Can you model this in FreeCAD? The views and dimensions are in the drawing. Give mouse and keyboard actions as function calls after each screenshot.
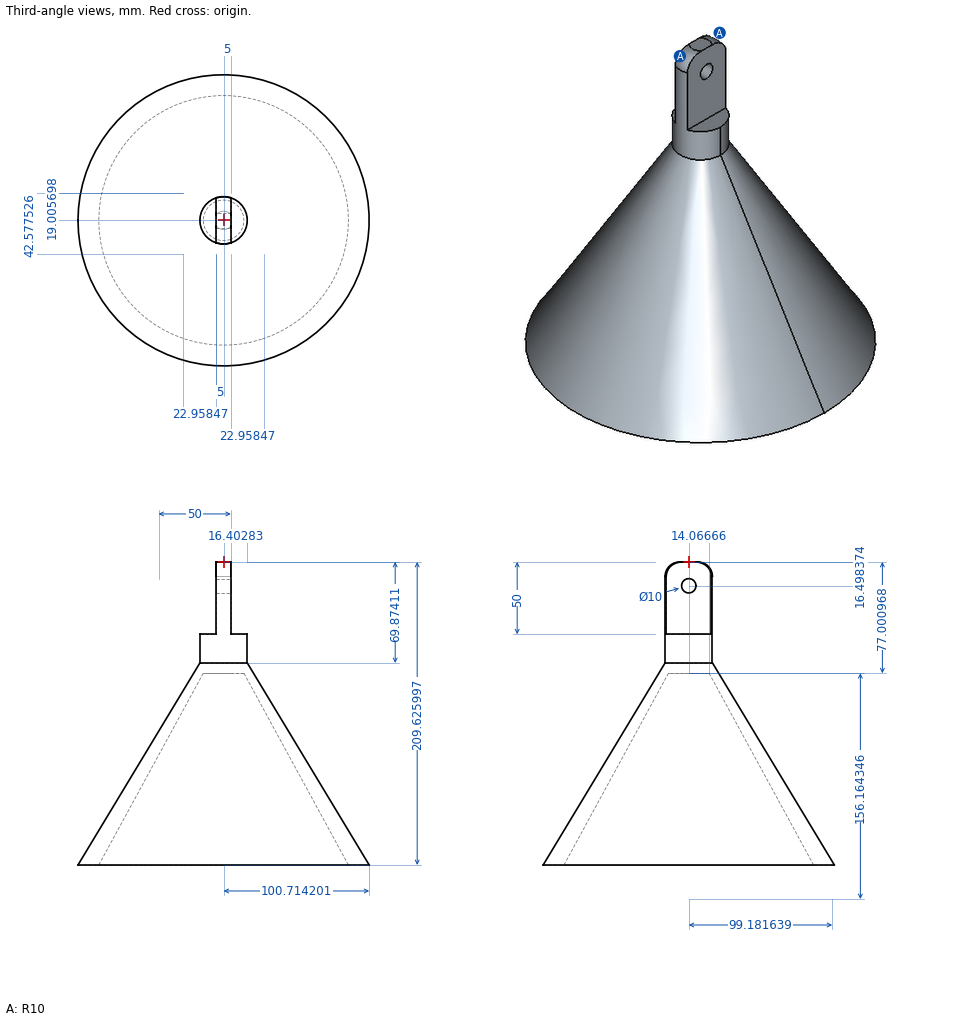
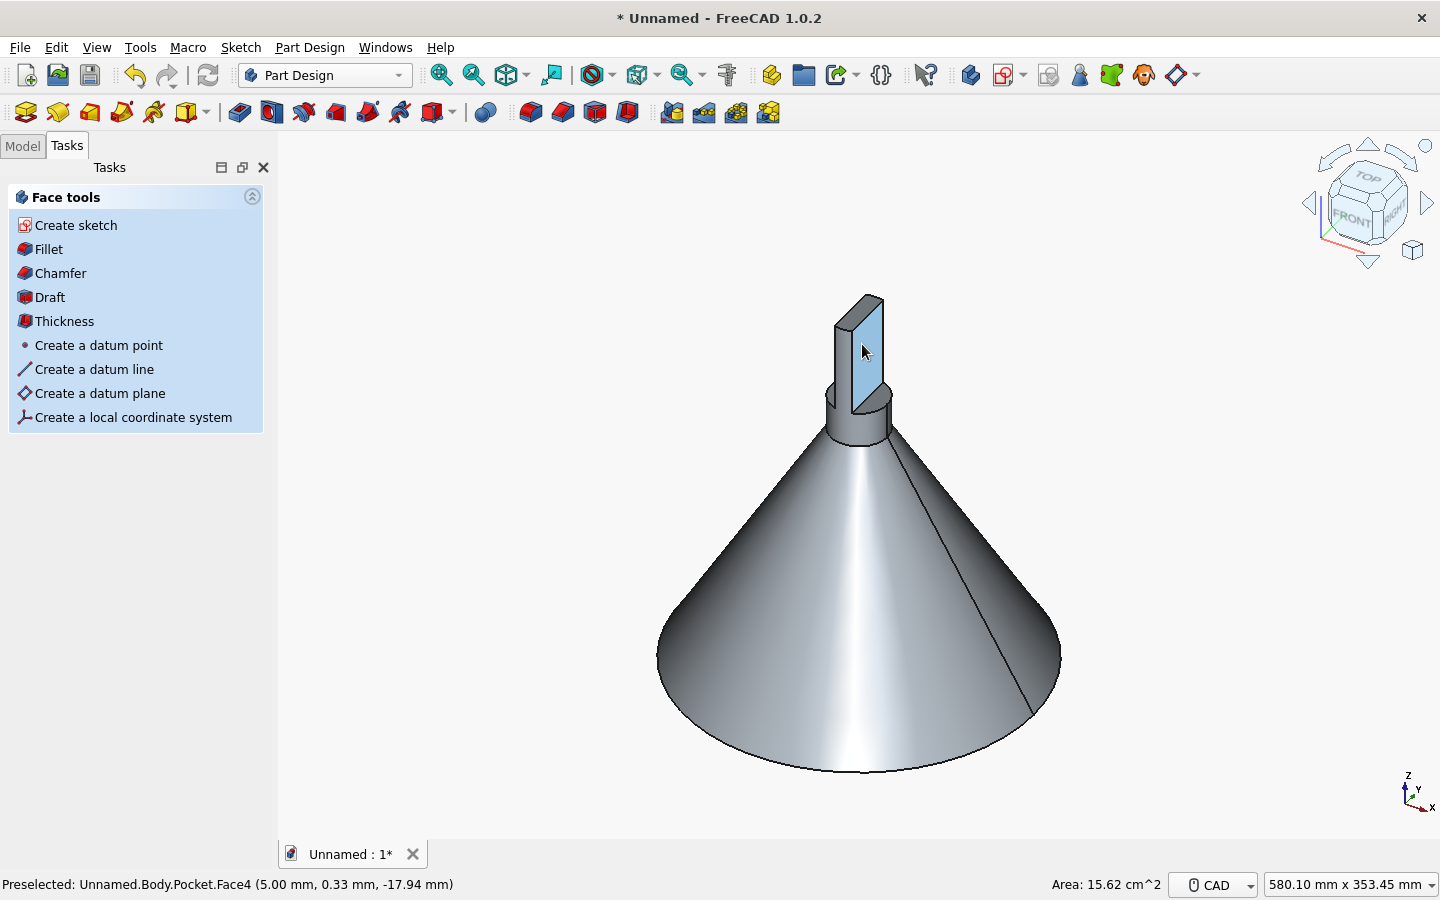
click(1004, 76)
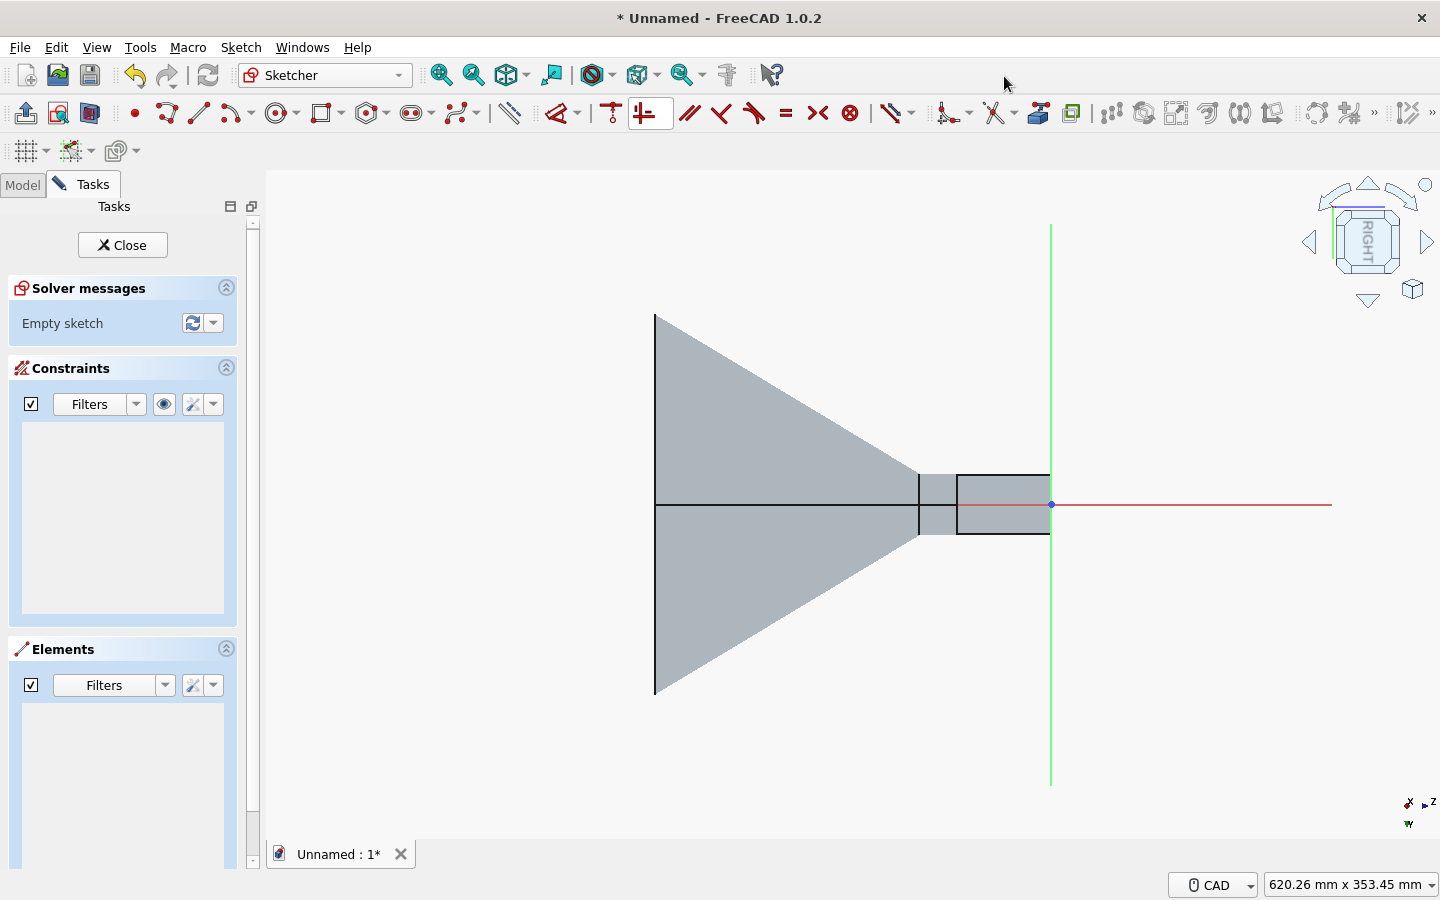
click(90, 114)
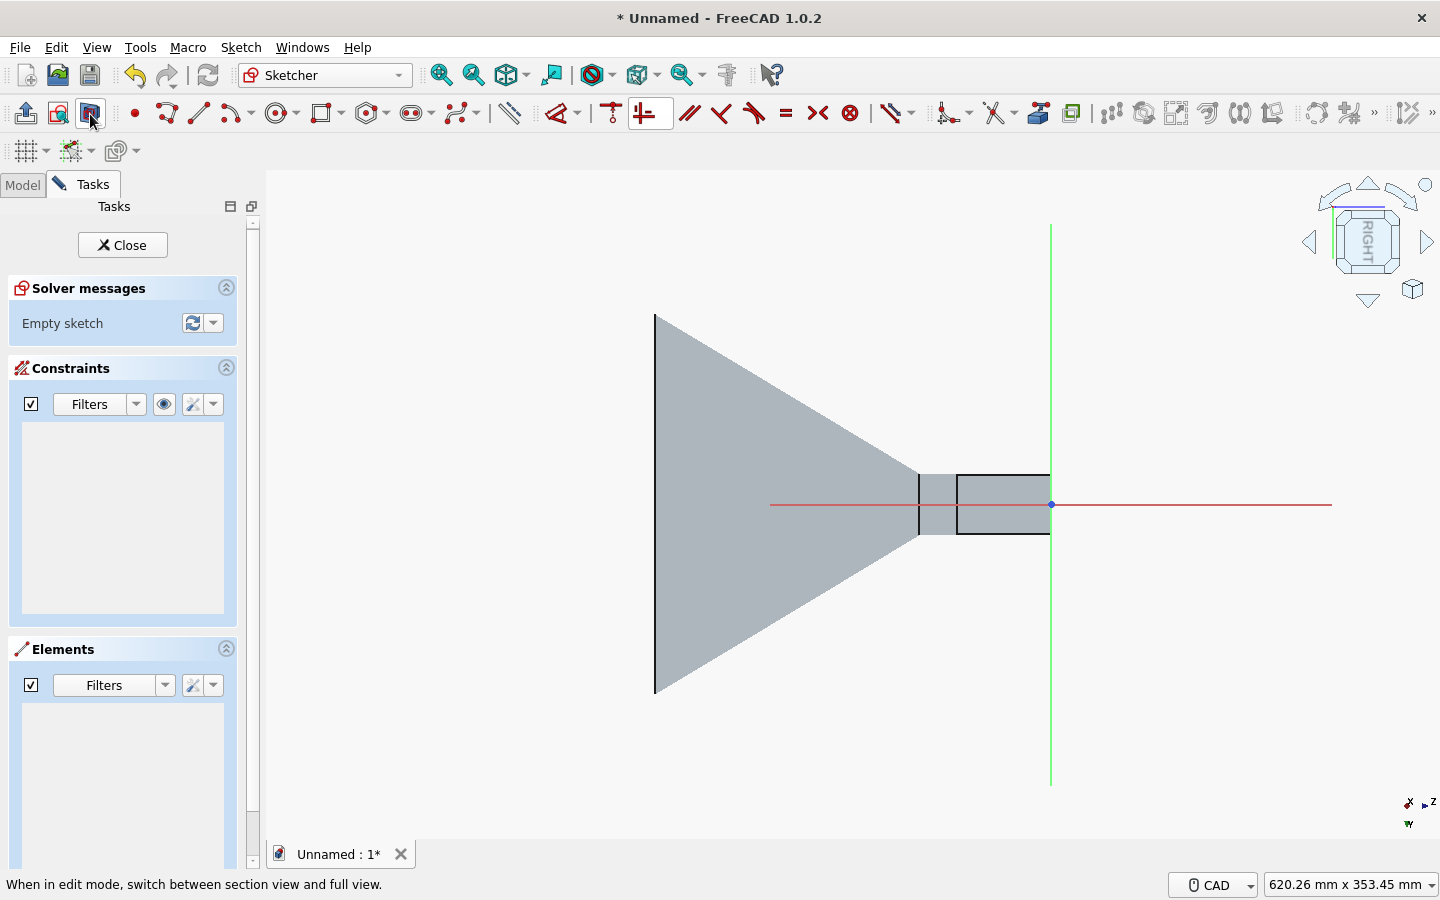
scroll(1047, 504, up, 14)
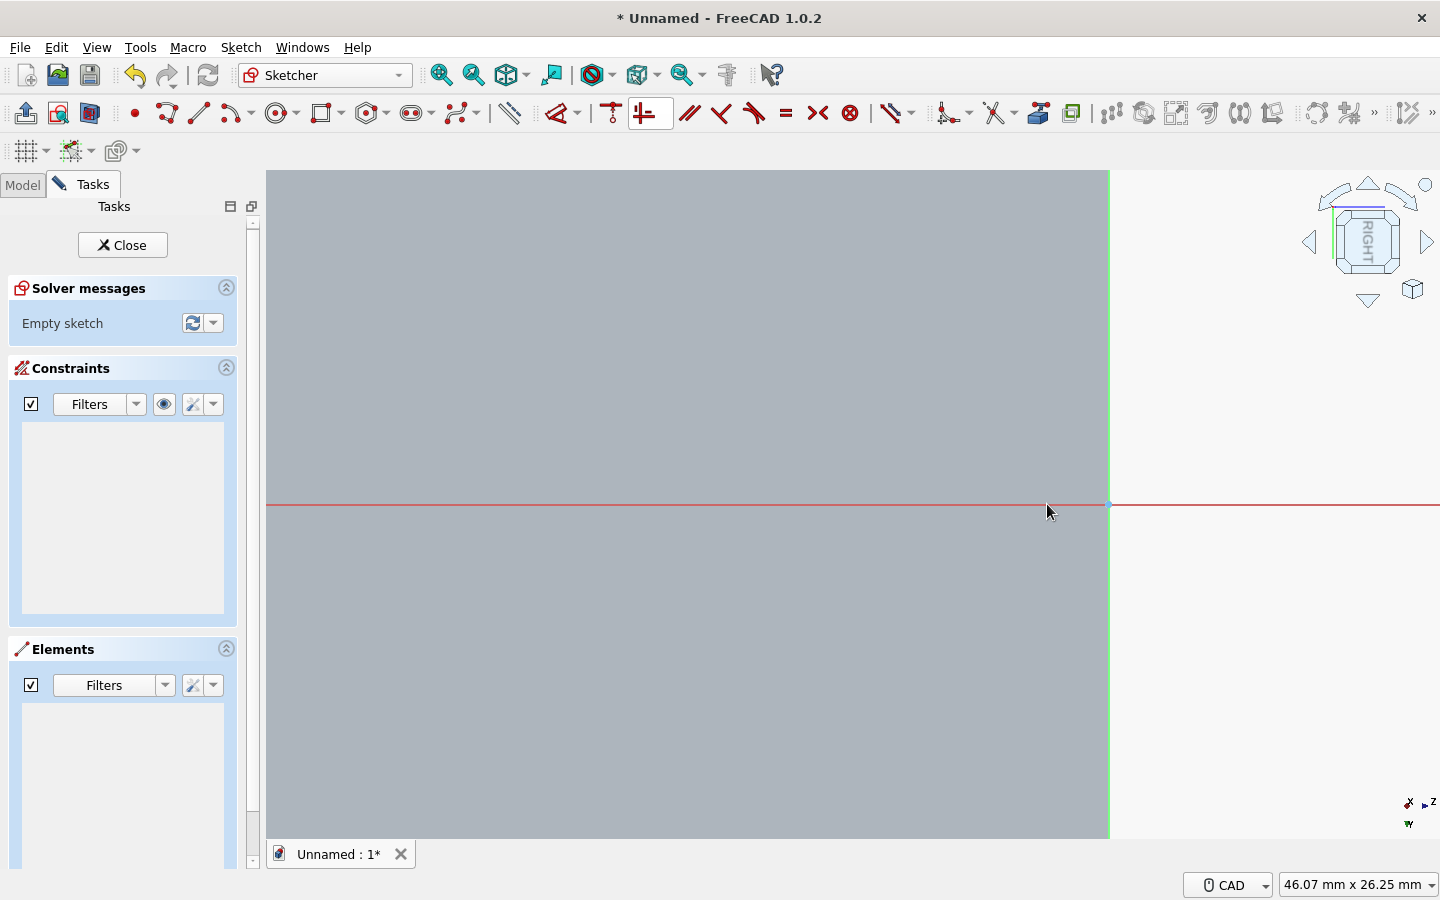
click(276, 114)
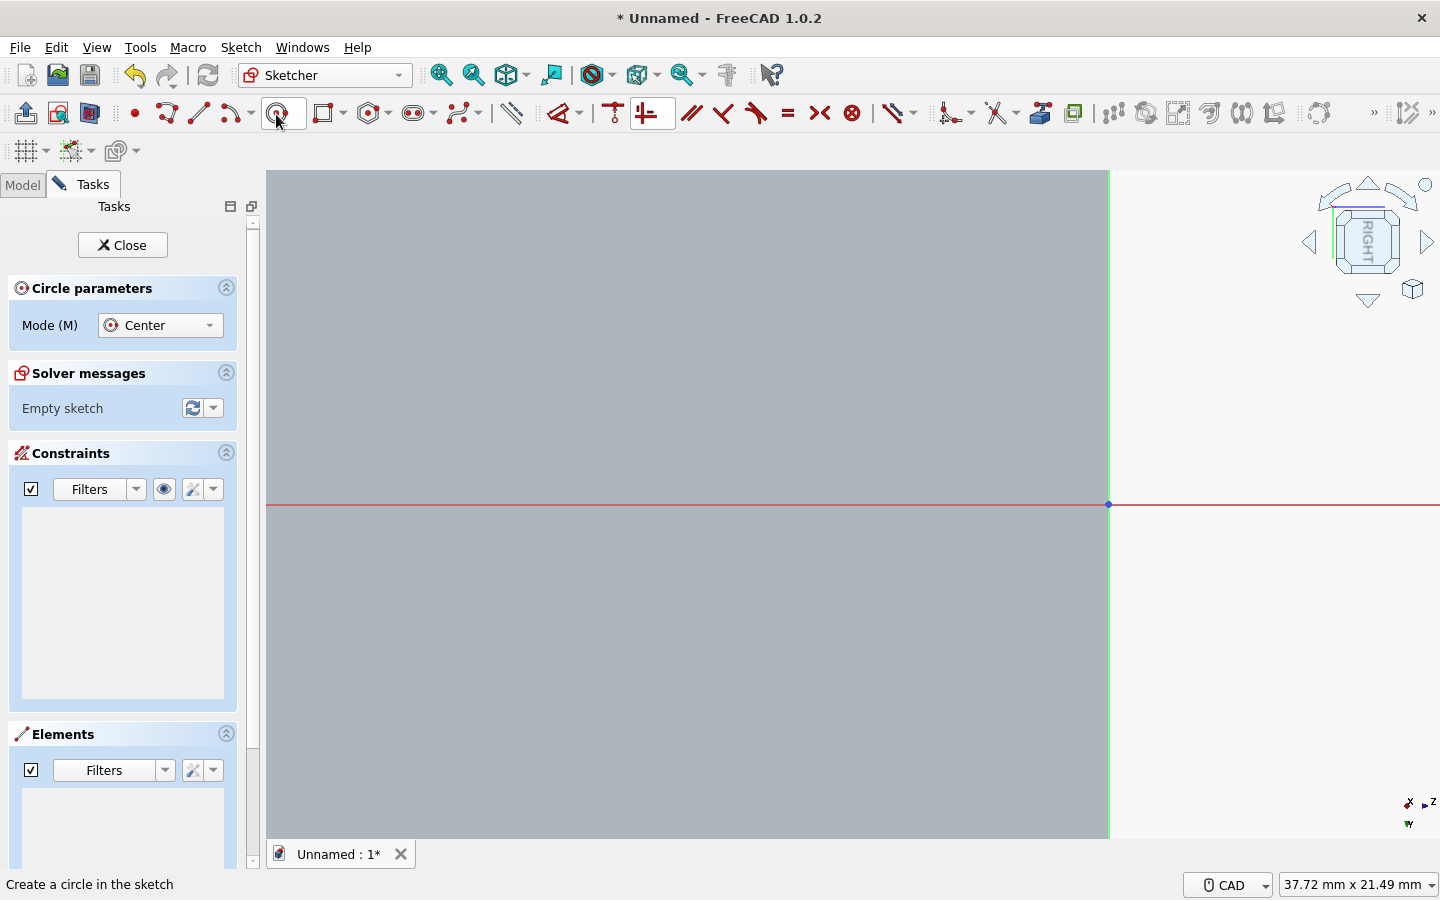
click(595, 504)
click(705, 394)
key(Escape)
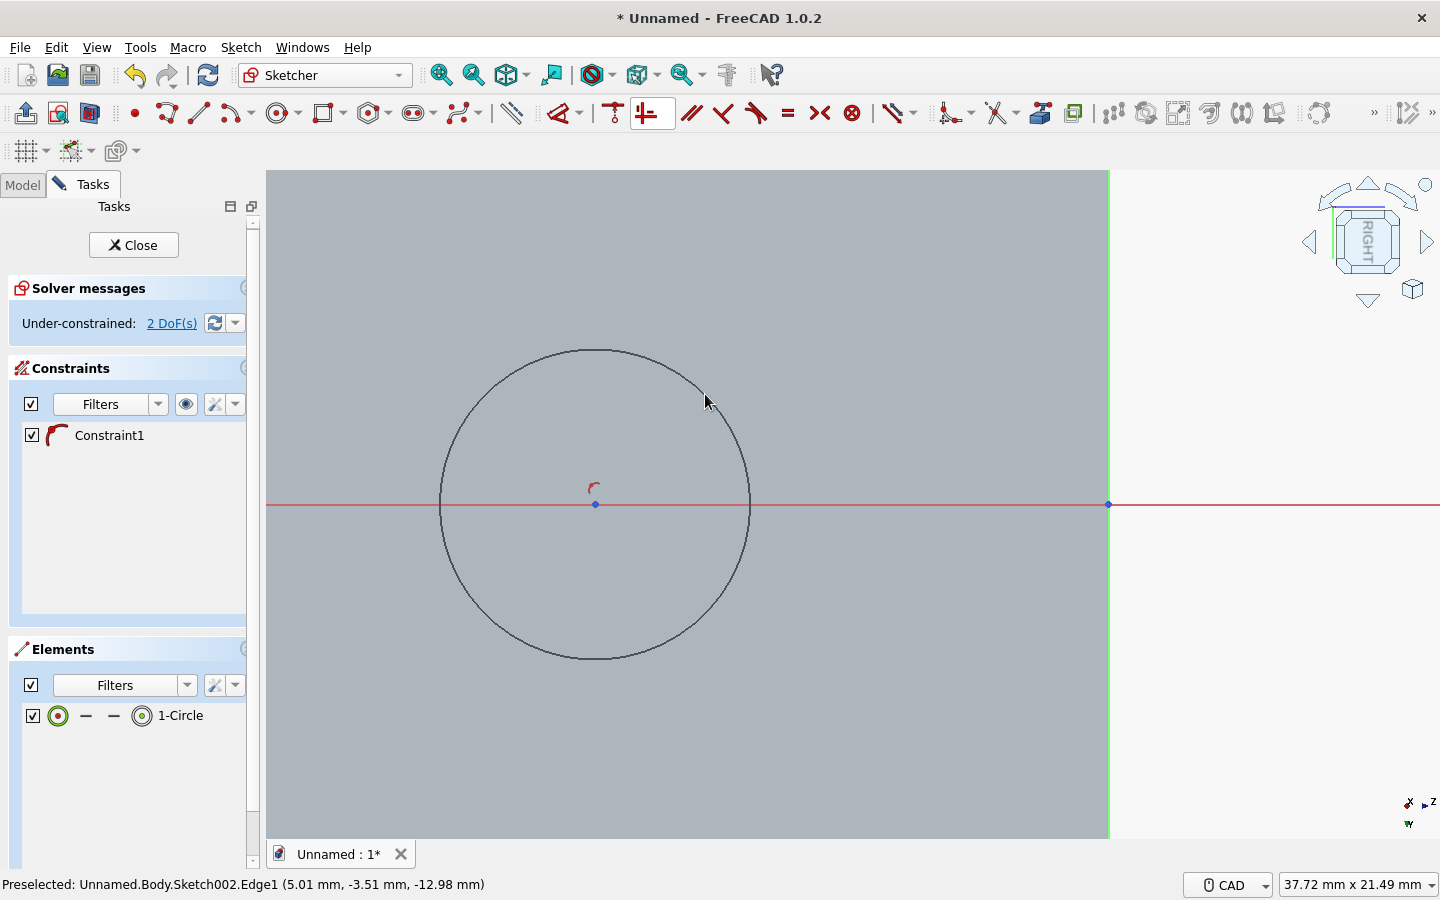
click(558, 114)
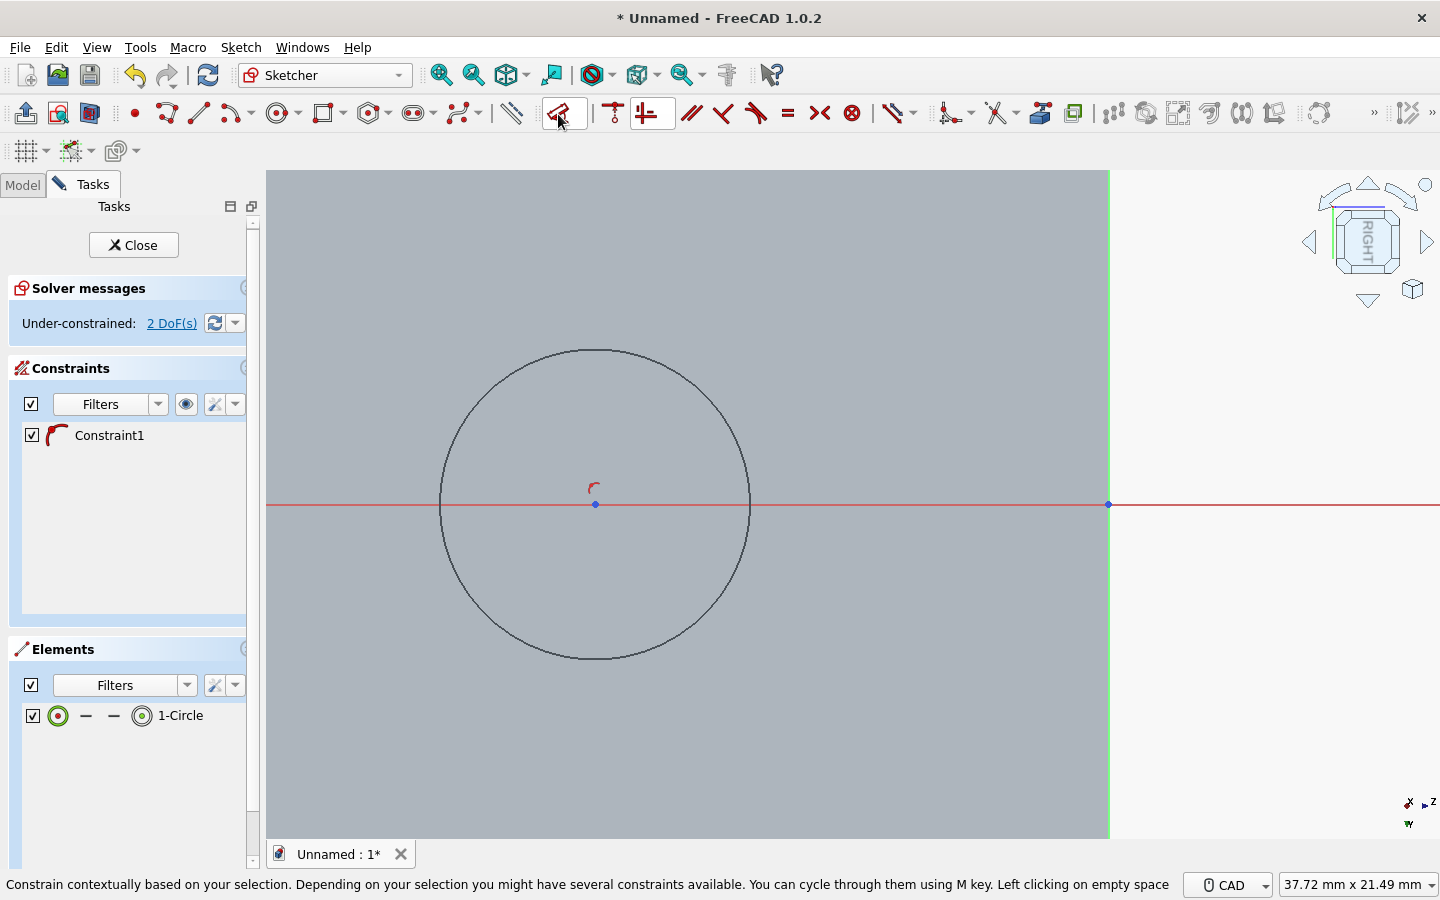
click(704, 394)
click(726, 371)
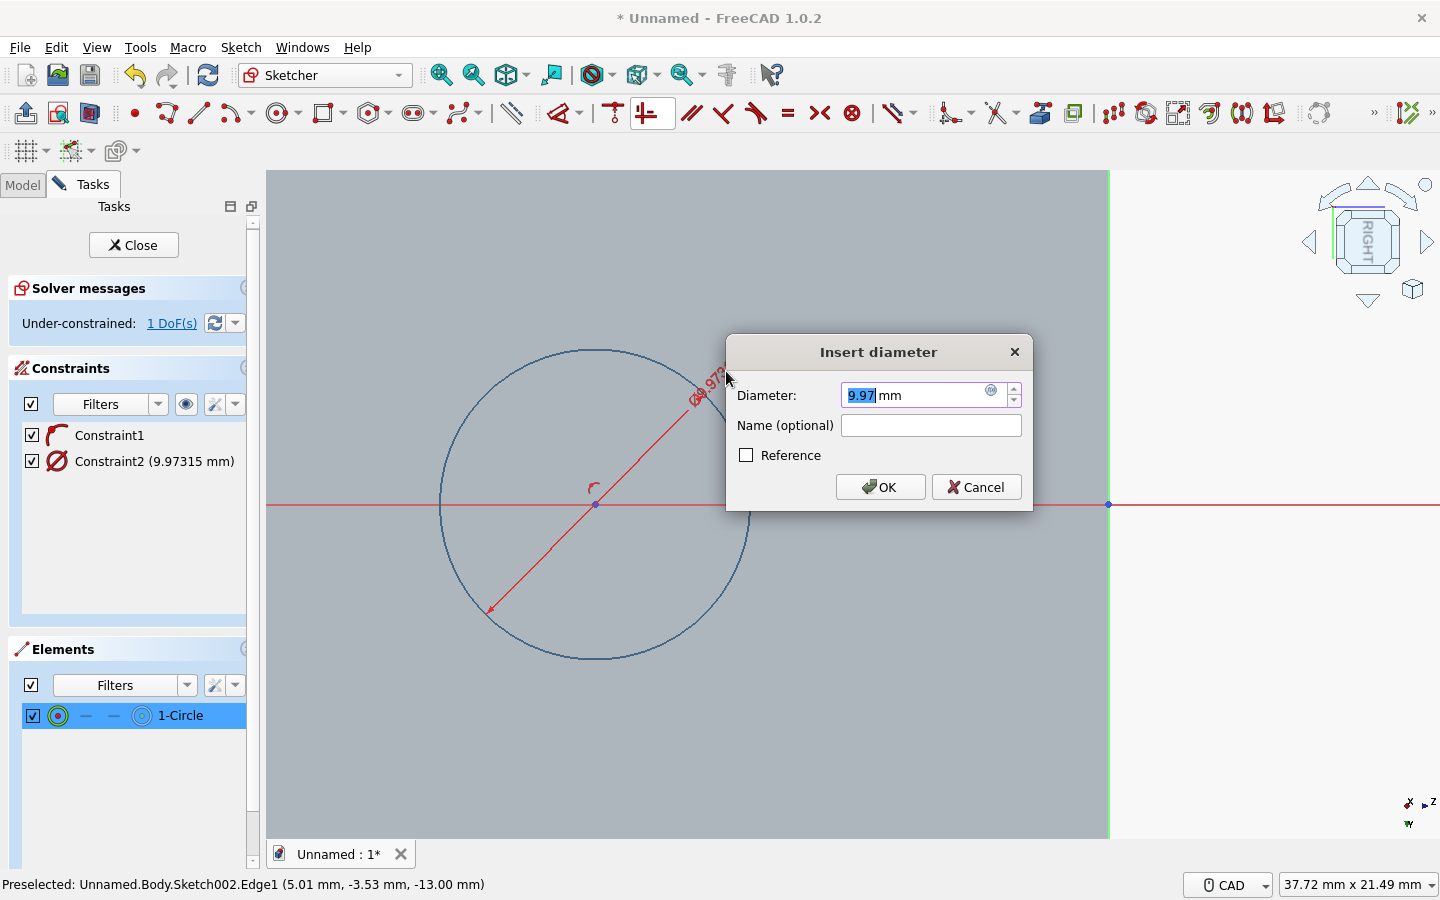
text(10)
key(Return)